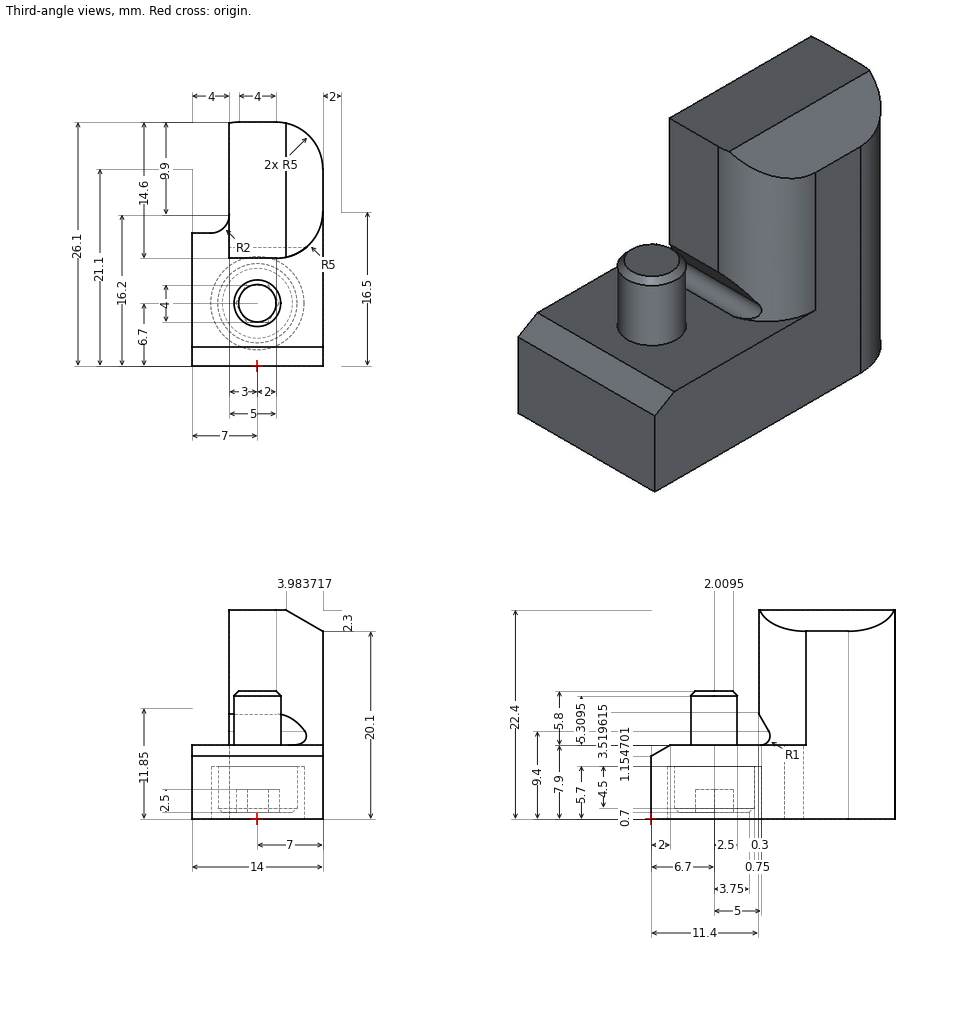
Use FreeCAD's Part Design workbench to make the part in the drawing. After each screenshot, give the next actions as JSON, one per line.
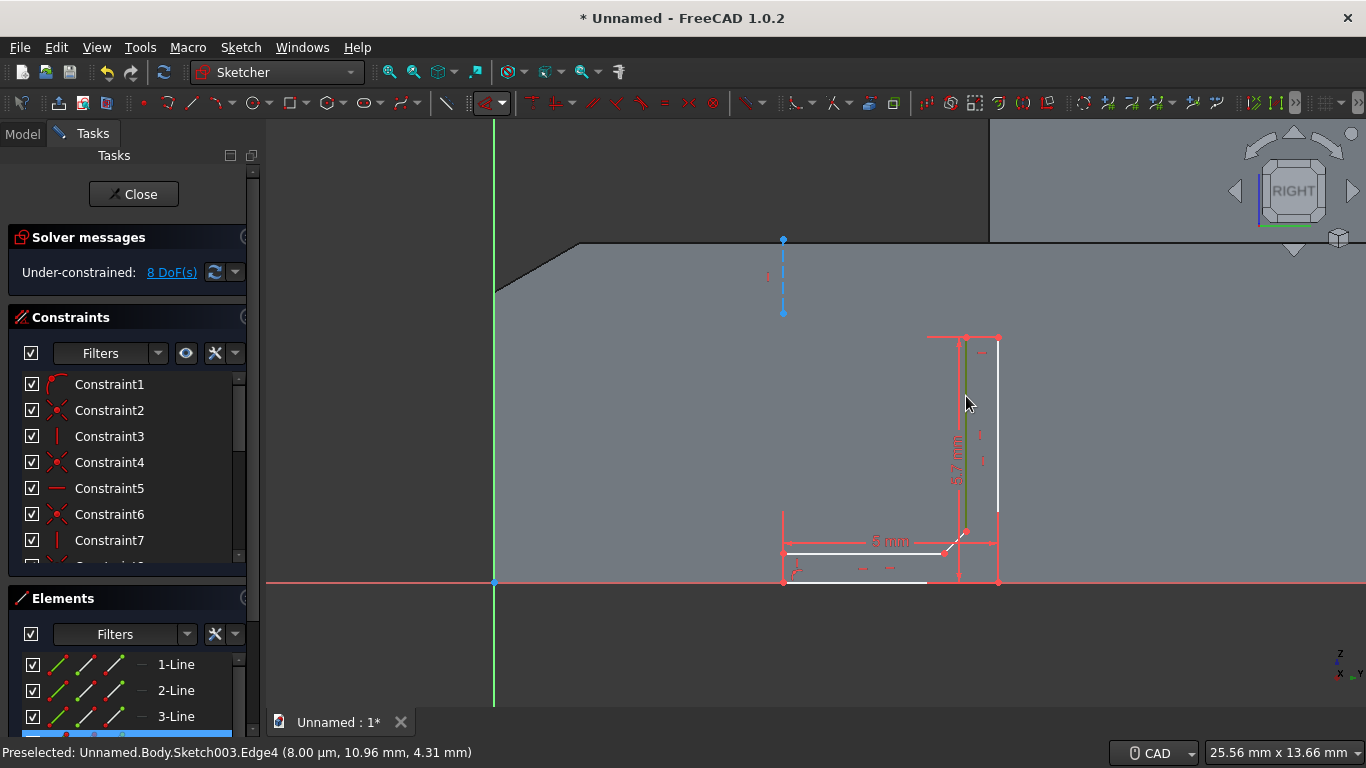
{"action": "key", "text": "i"}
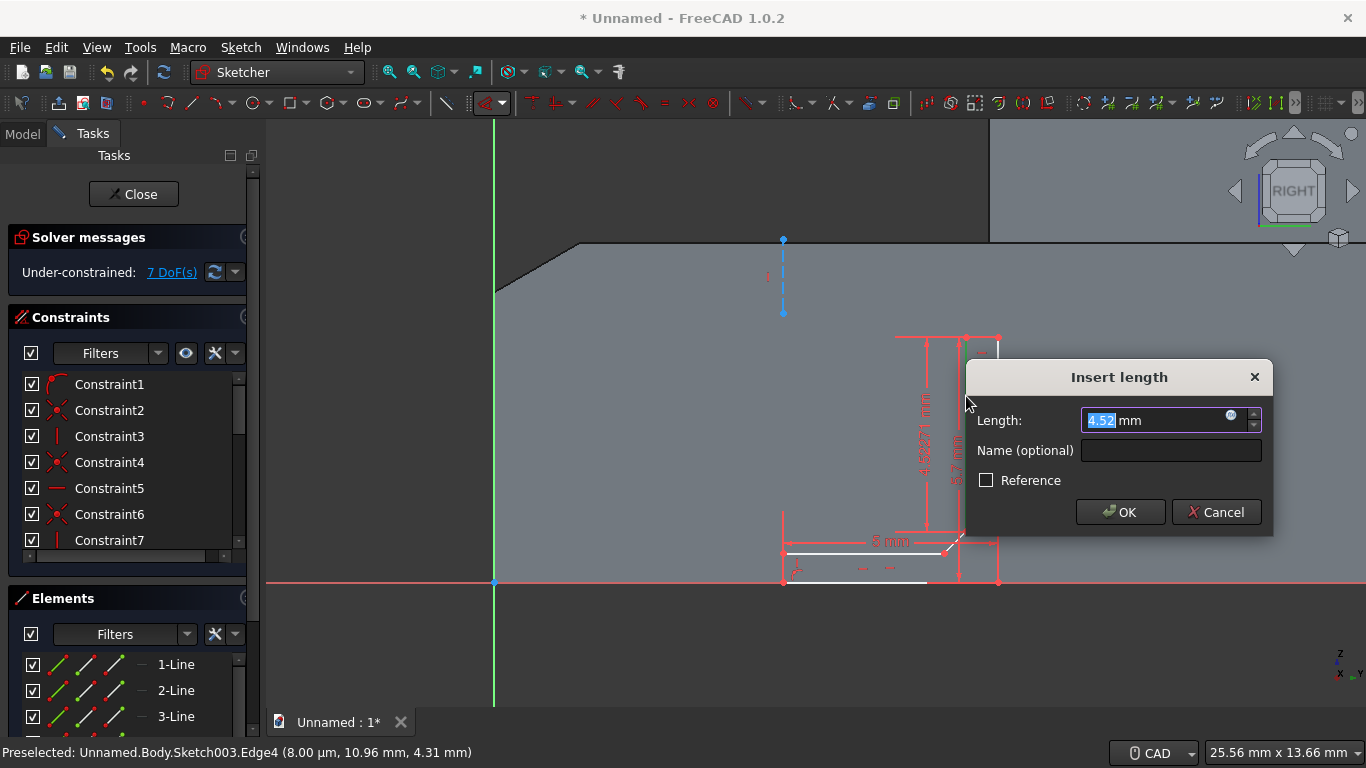
{"action": "type", "text": "4.5"}
{"action": "key", "text": "Return"}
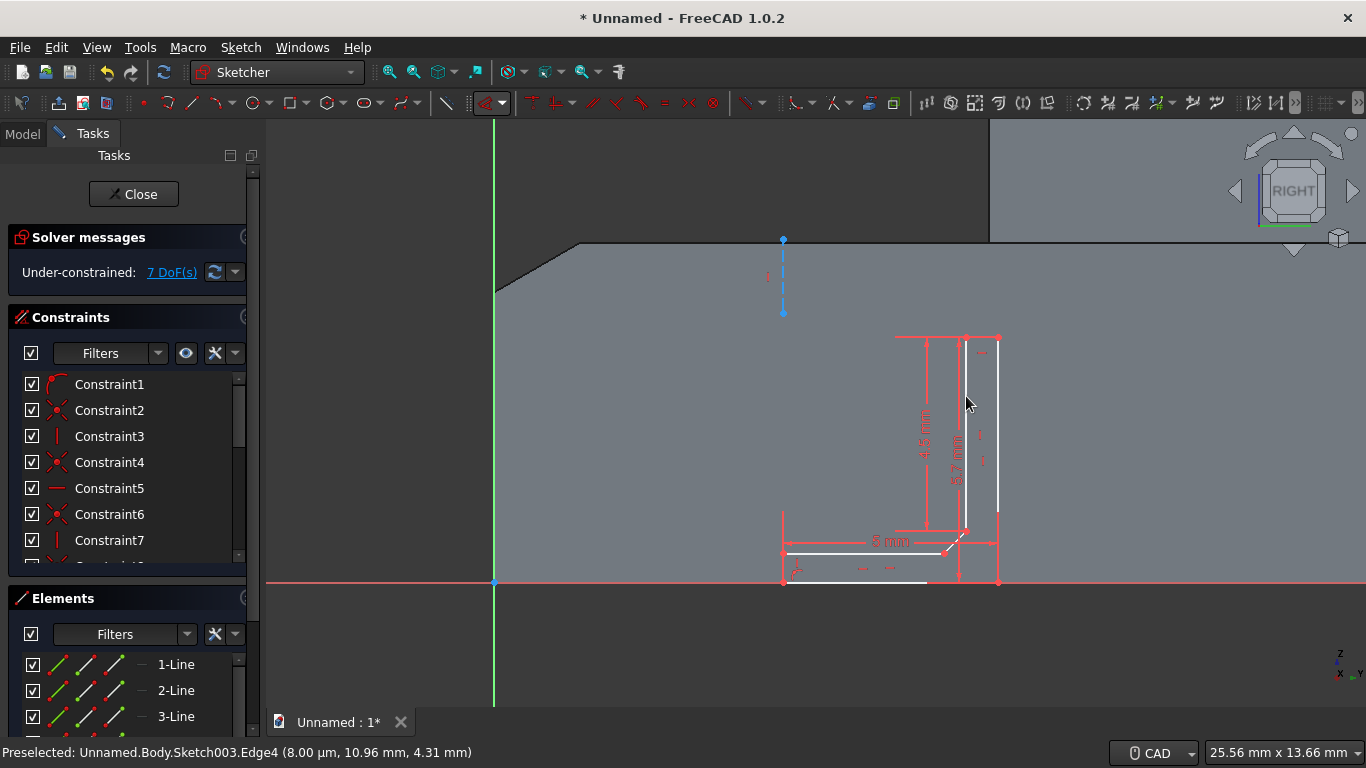
{"action": "scroll", "coordinate": [783, 565], "scroll_direction": "up", "scroll_amount": 2}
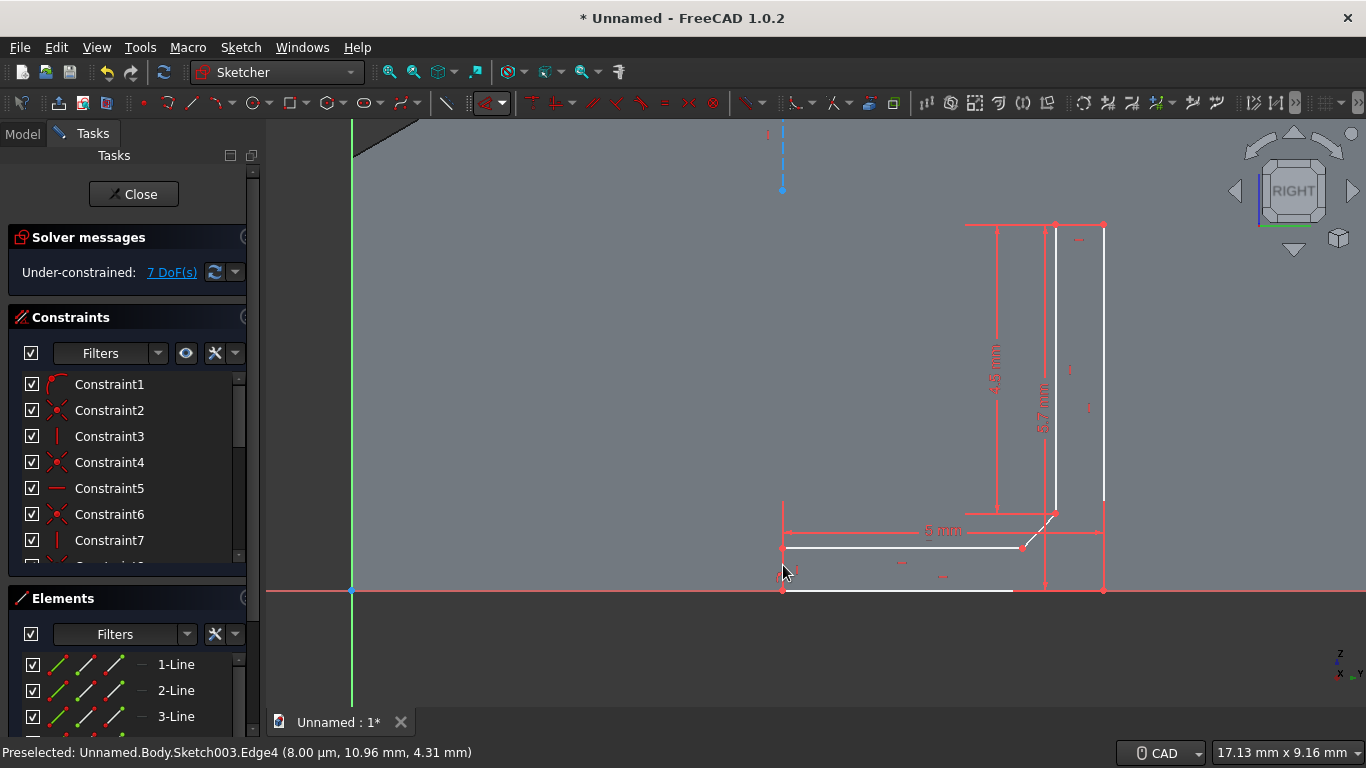
{"action": "left_click", "coordinate": [783, 565]}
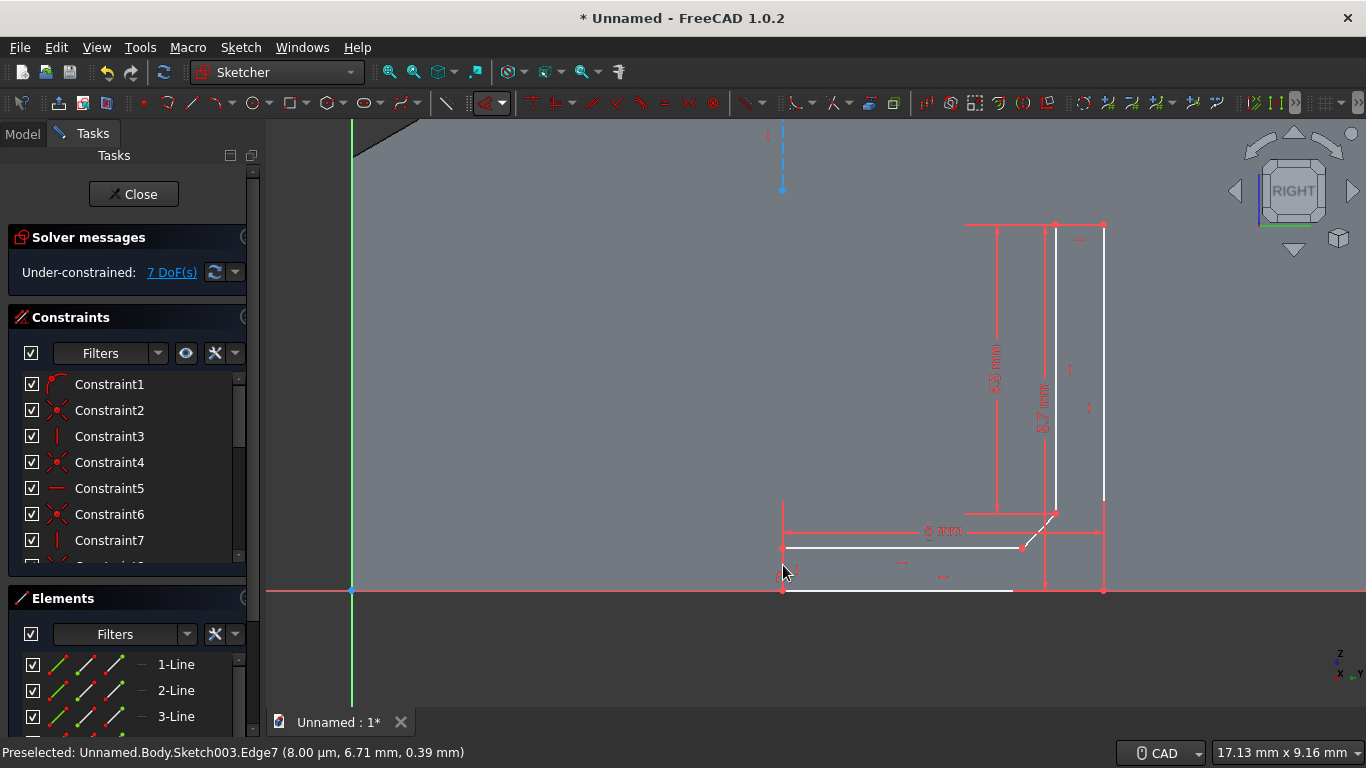
{"action": "left_click", "coordinate": [504, 104]}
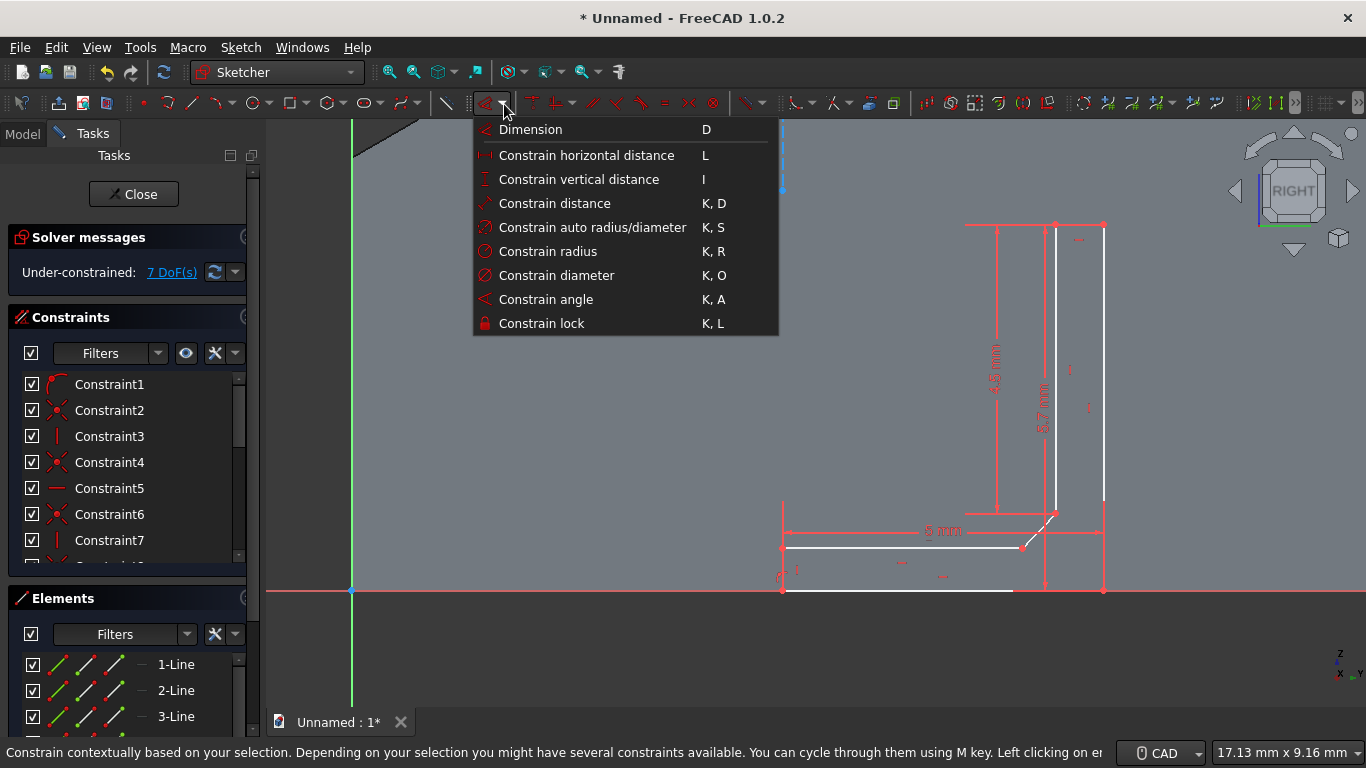
{"action": "left_click", "coordinate": [626, 179]}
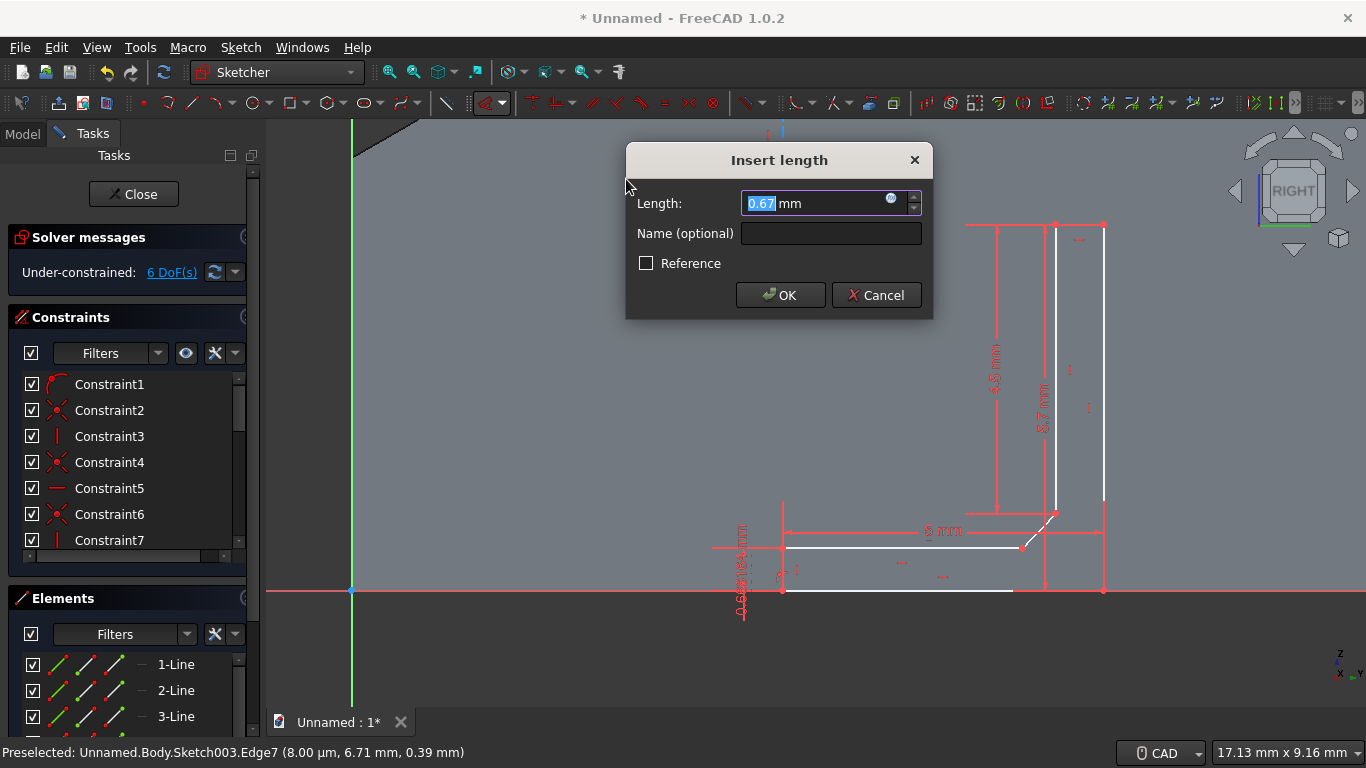
{"action": "type", "text": "0.7"}
{"action": "key", "text": "Return"}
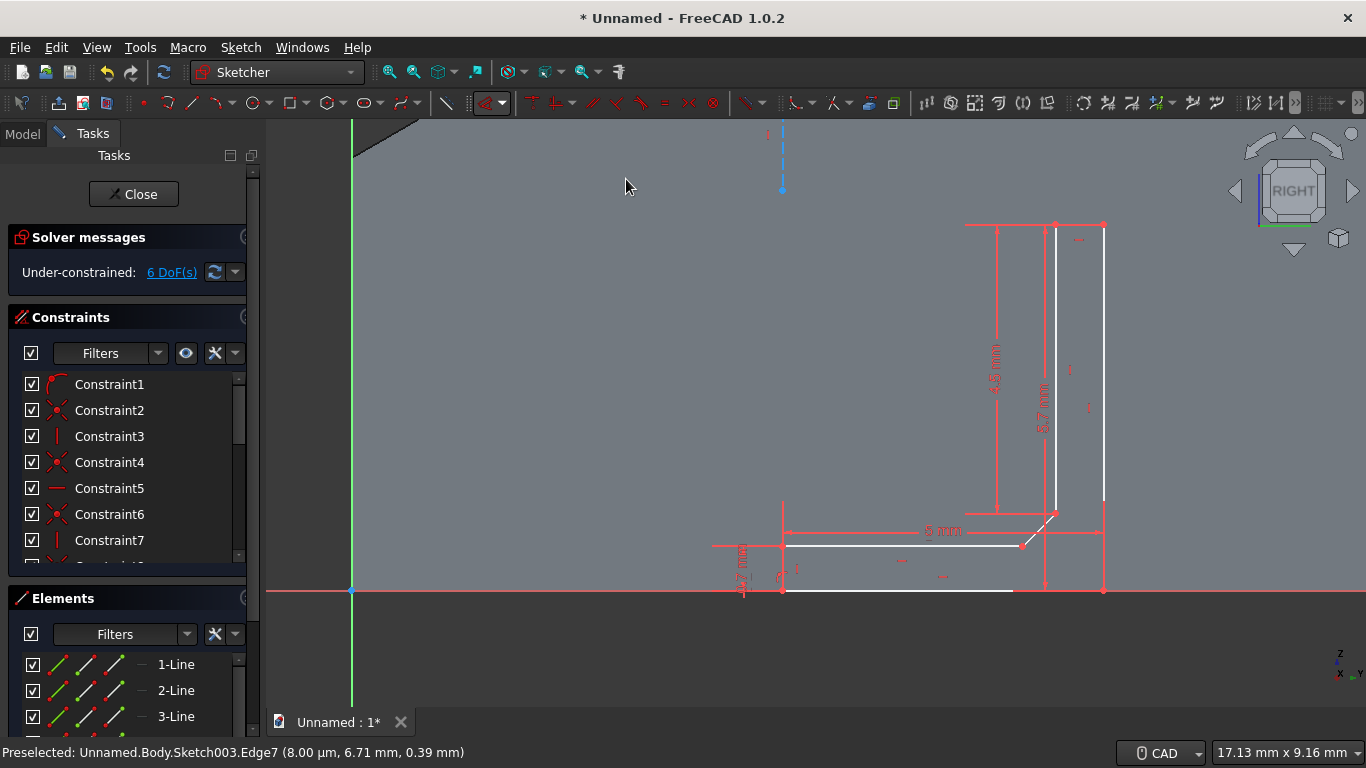
{"action": "left_click", "coordinate": [1089, 225]}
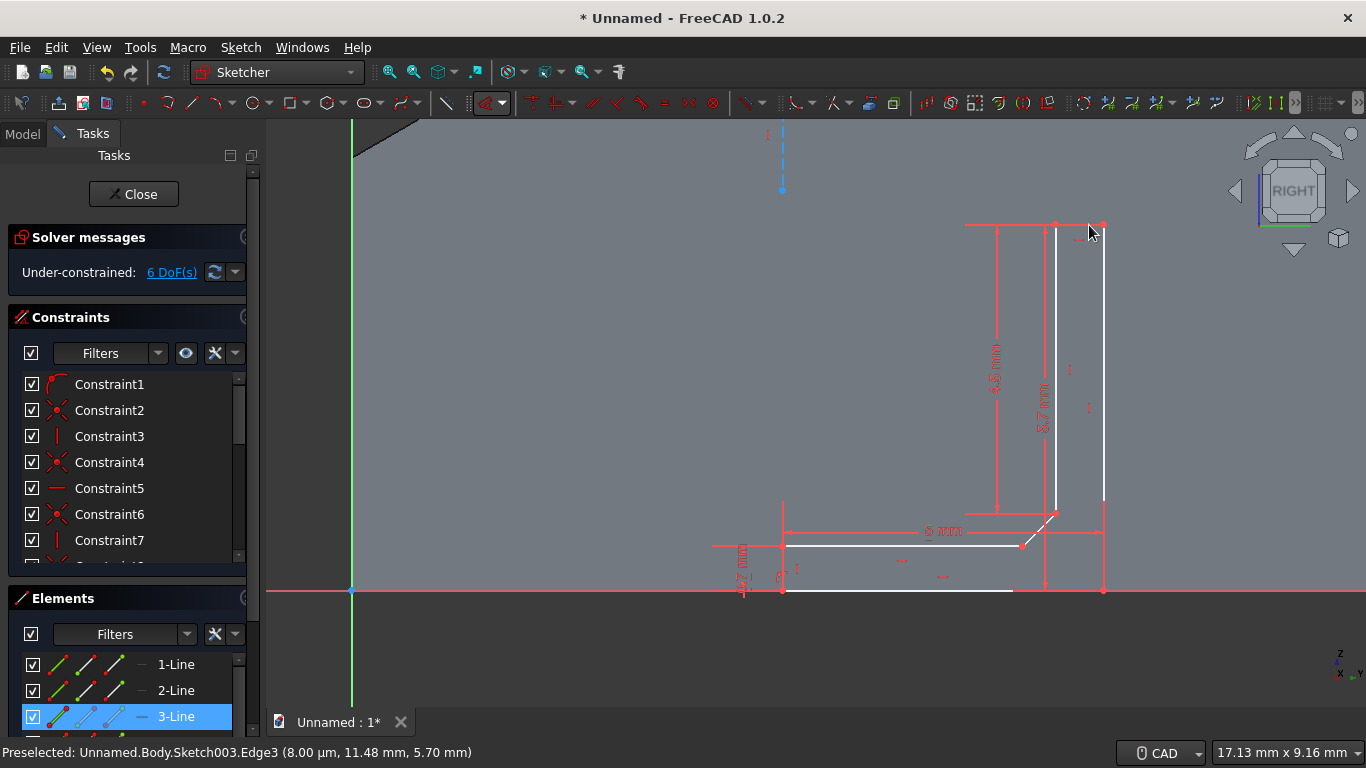
{"action": "left_click", "coordinate": [504, 104]}